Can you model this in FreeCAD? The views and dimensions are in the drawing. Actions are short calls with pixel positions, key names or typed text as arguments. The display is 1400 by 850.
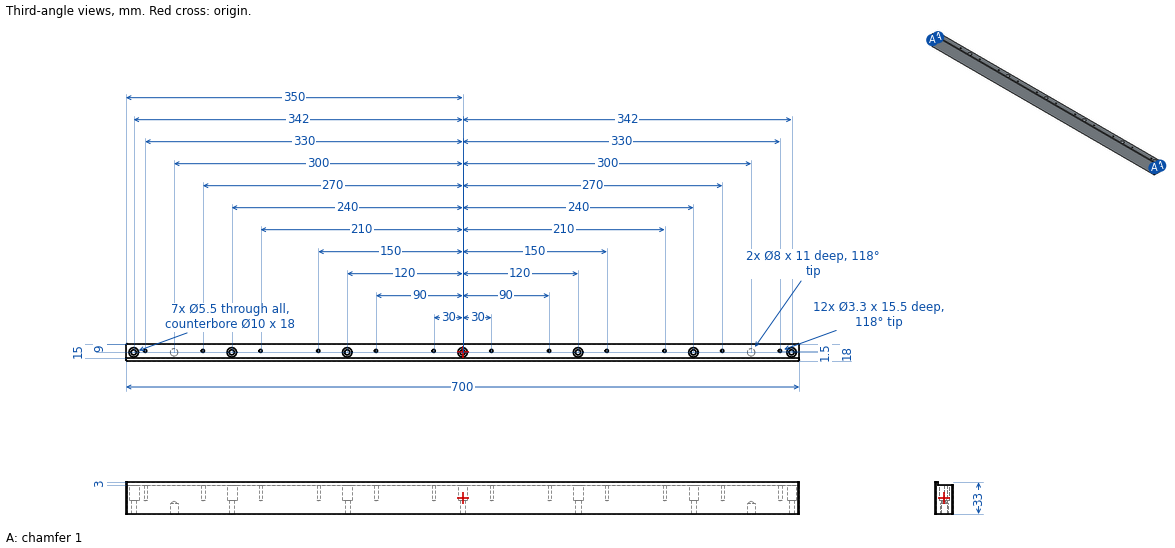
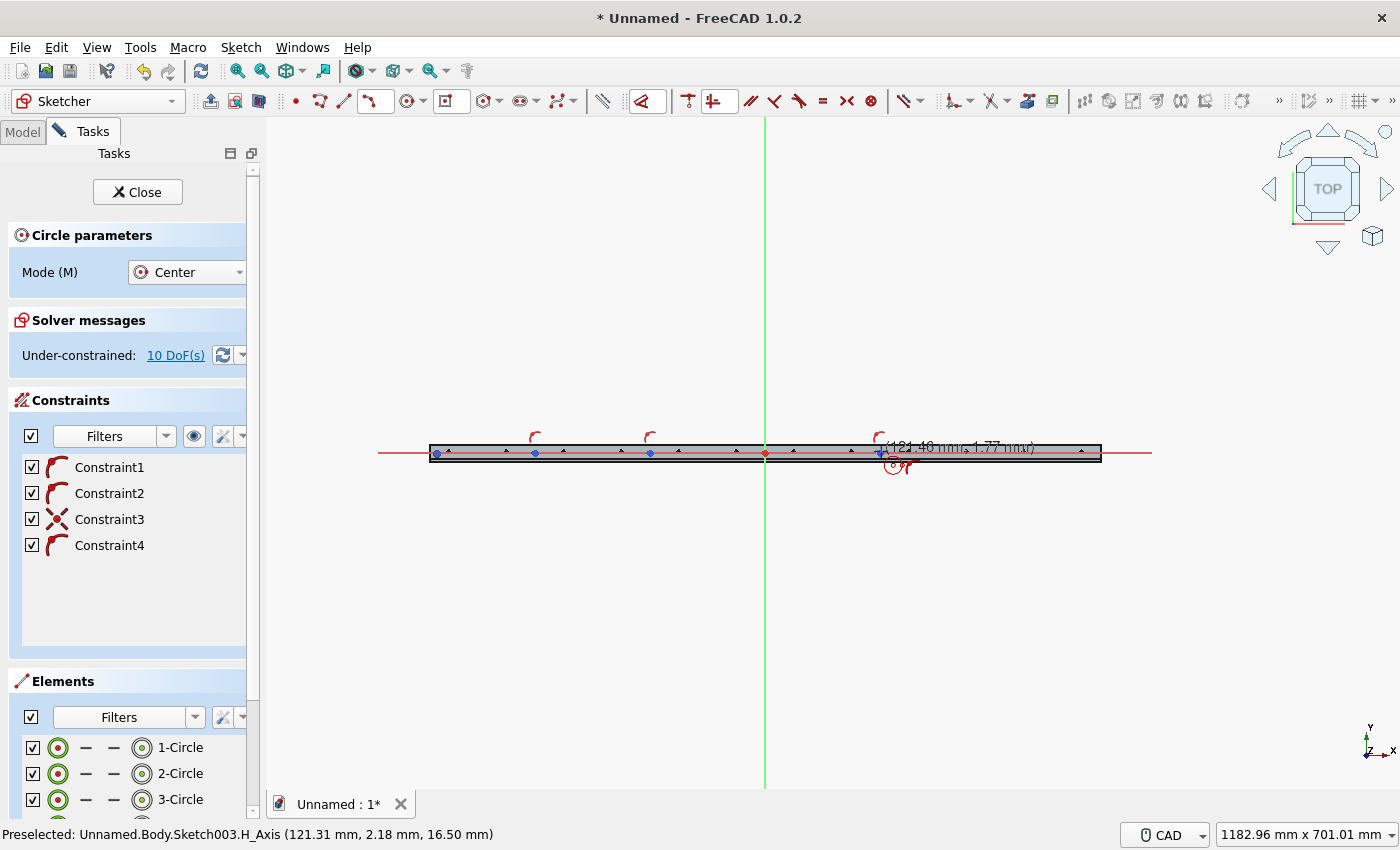
scroll(995, 453, up, 11)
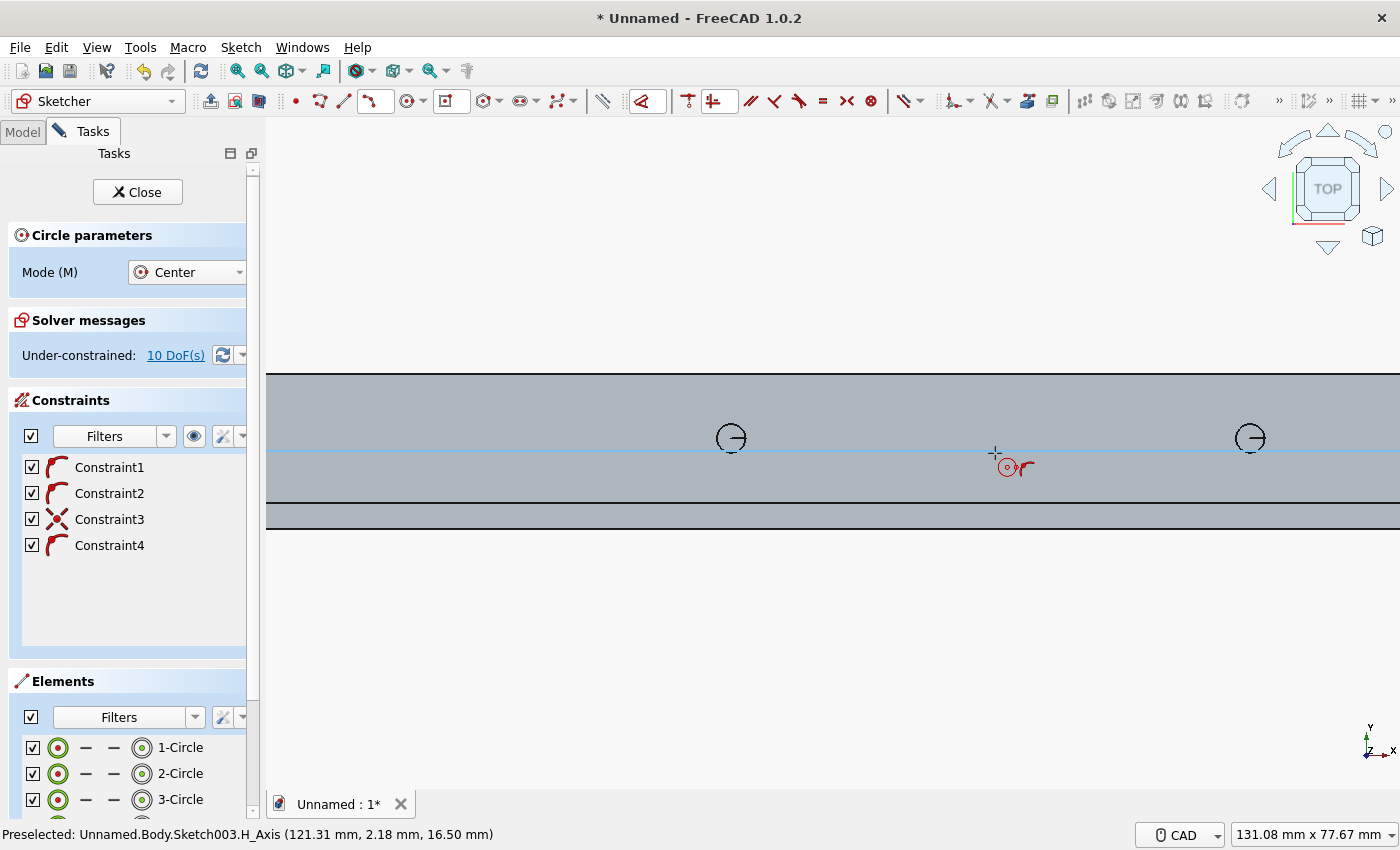
scroll(995, 453, down, 11)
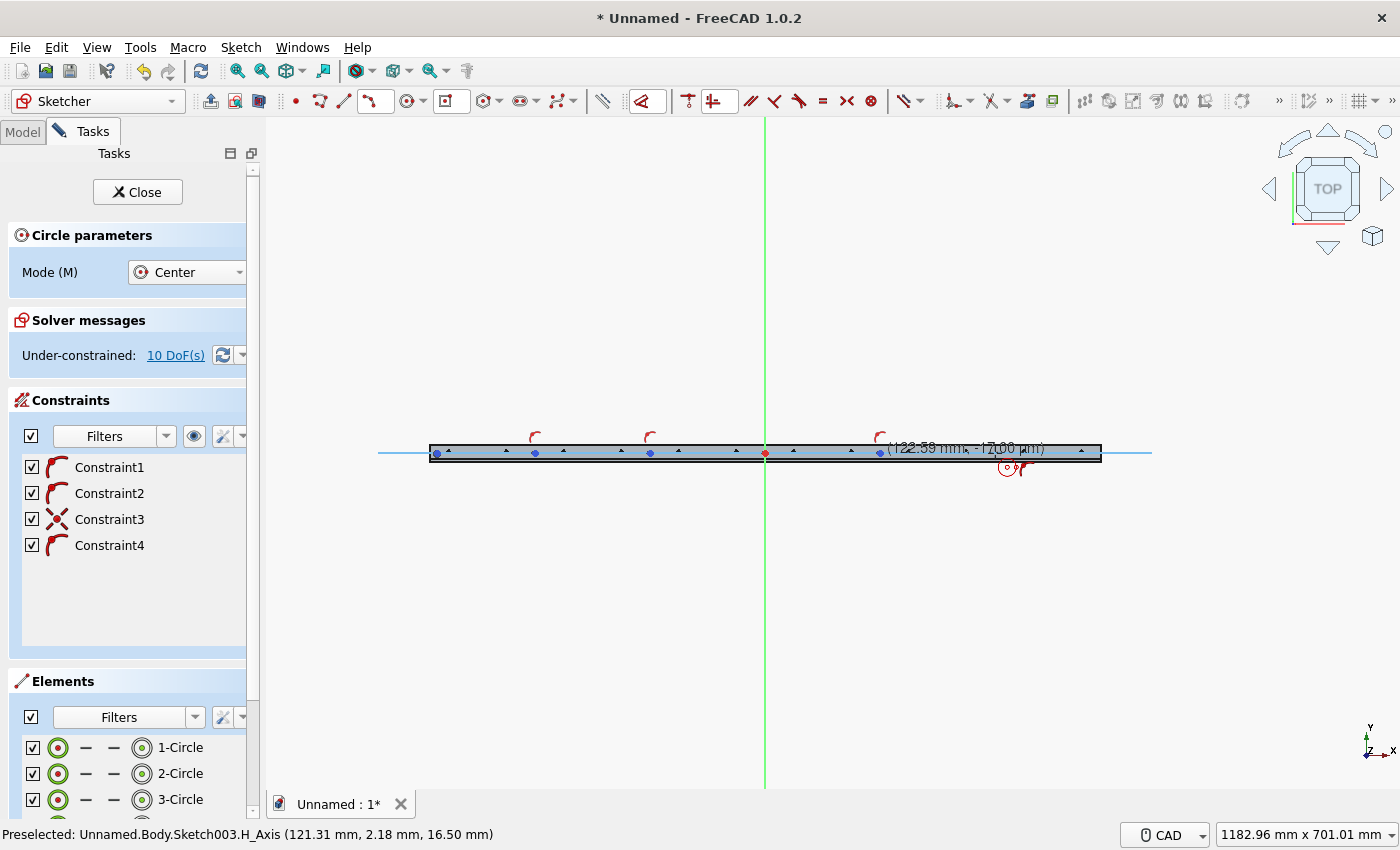
click(995, 453)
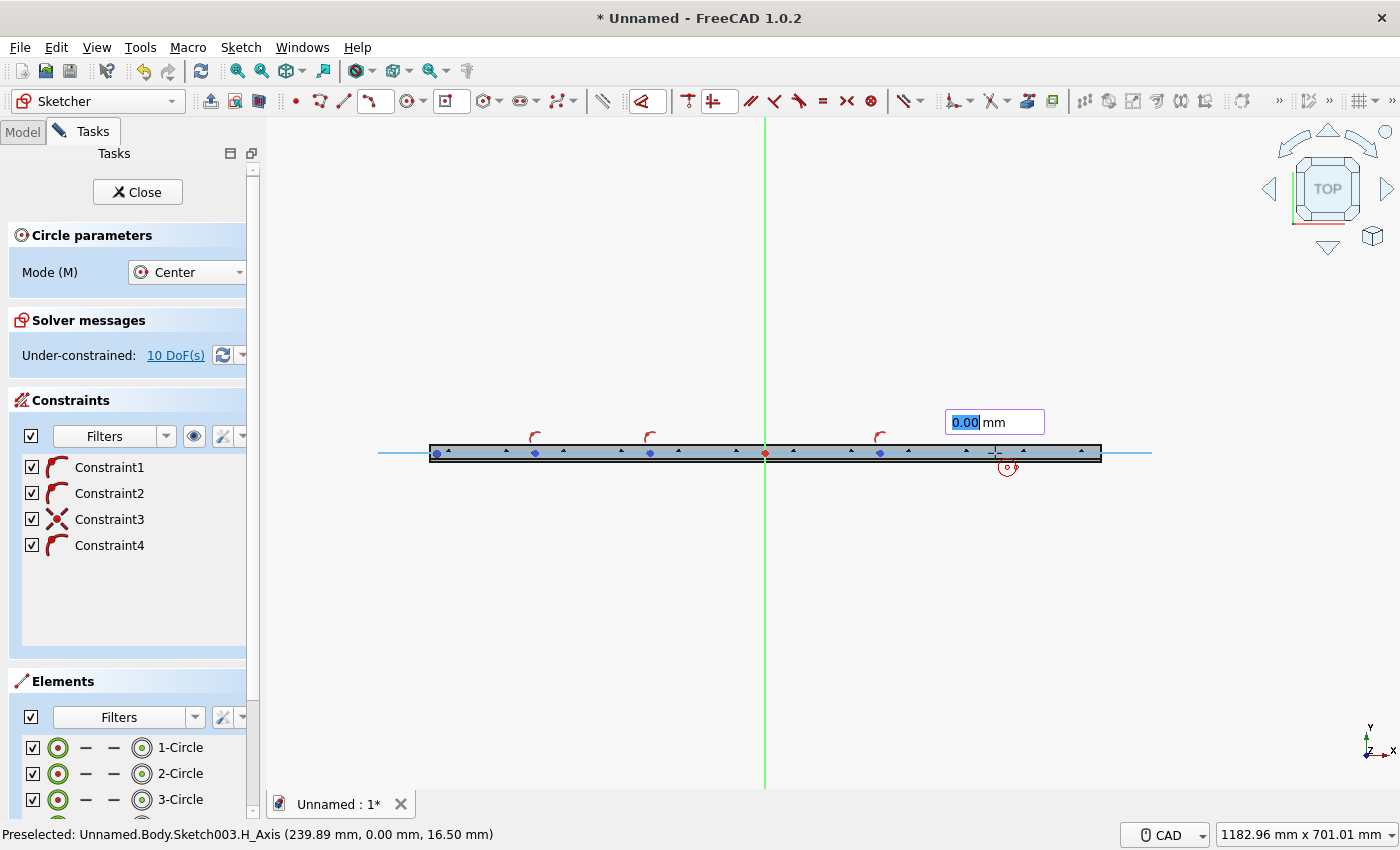
scroll(996, 451, up, 10)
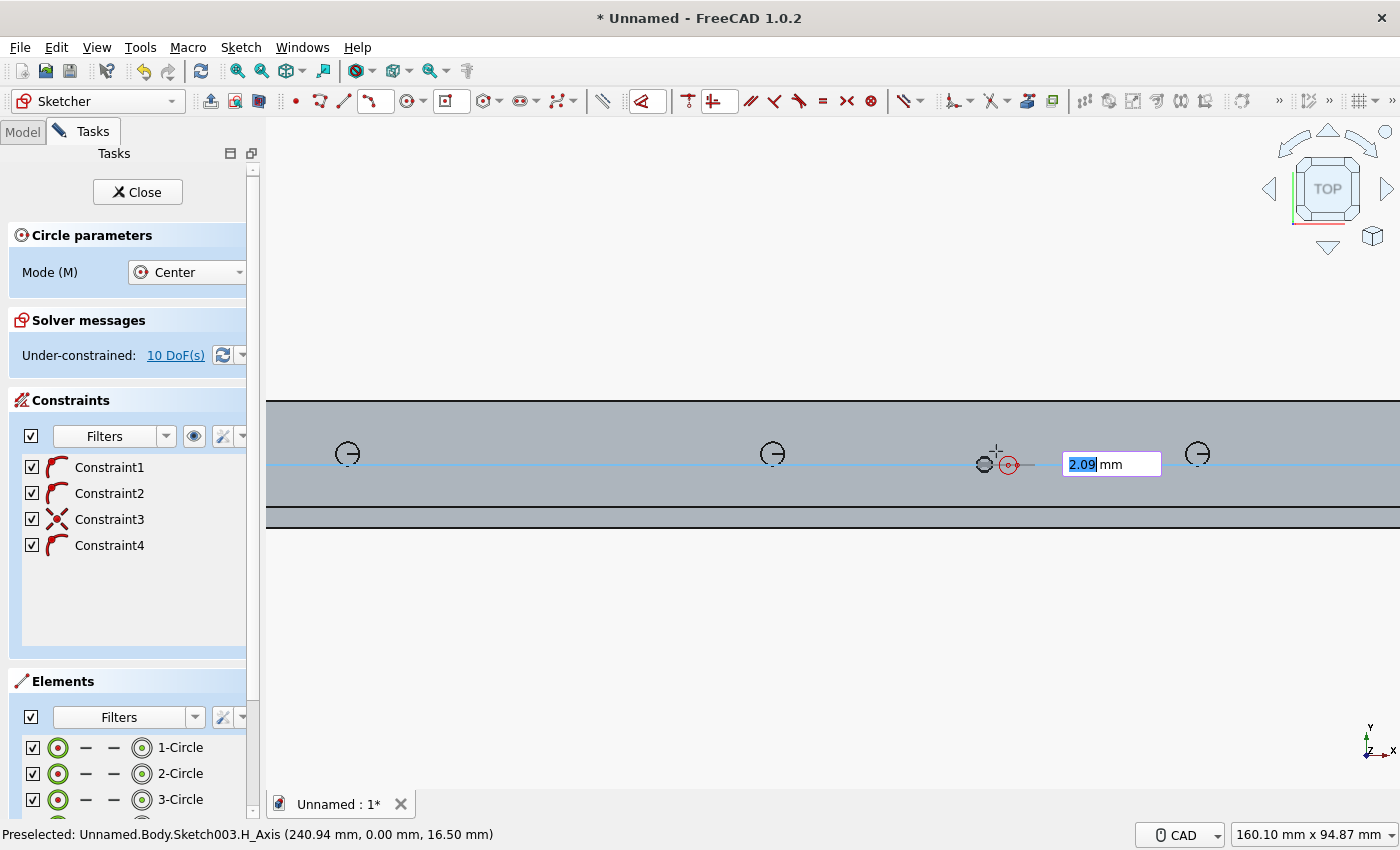
click(992, 446)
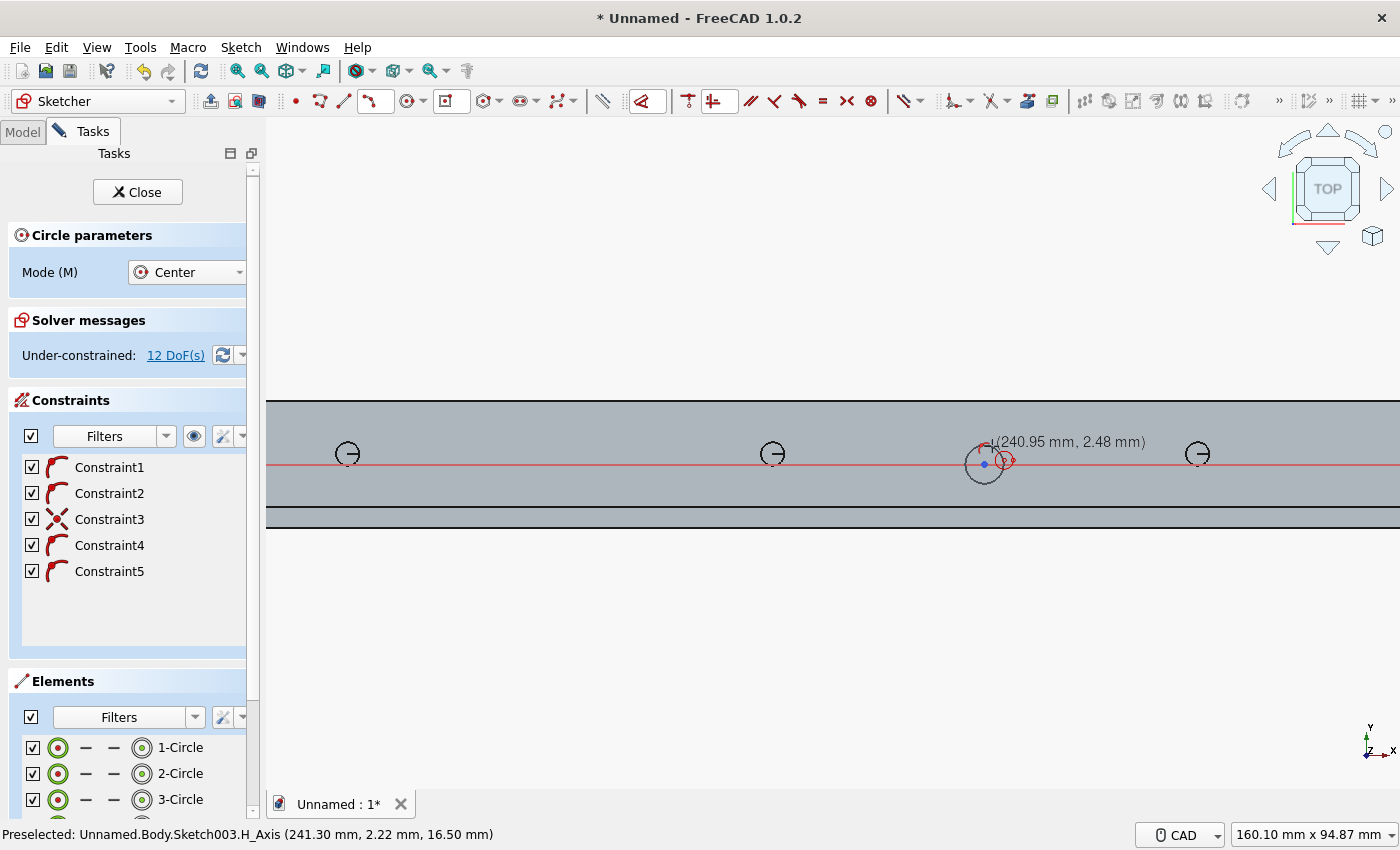
scroll(996, 451, down, 10)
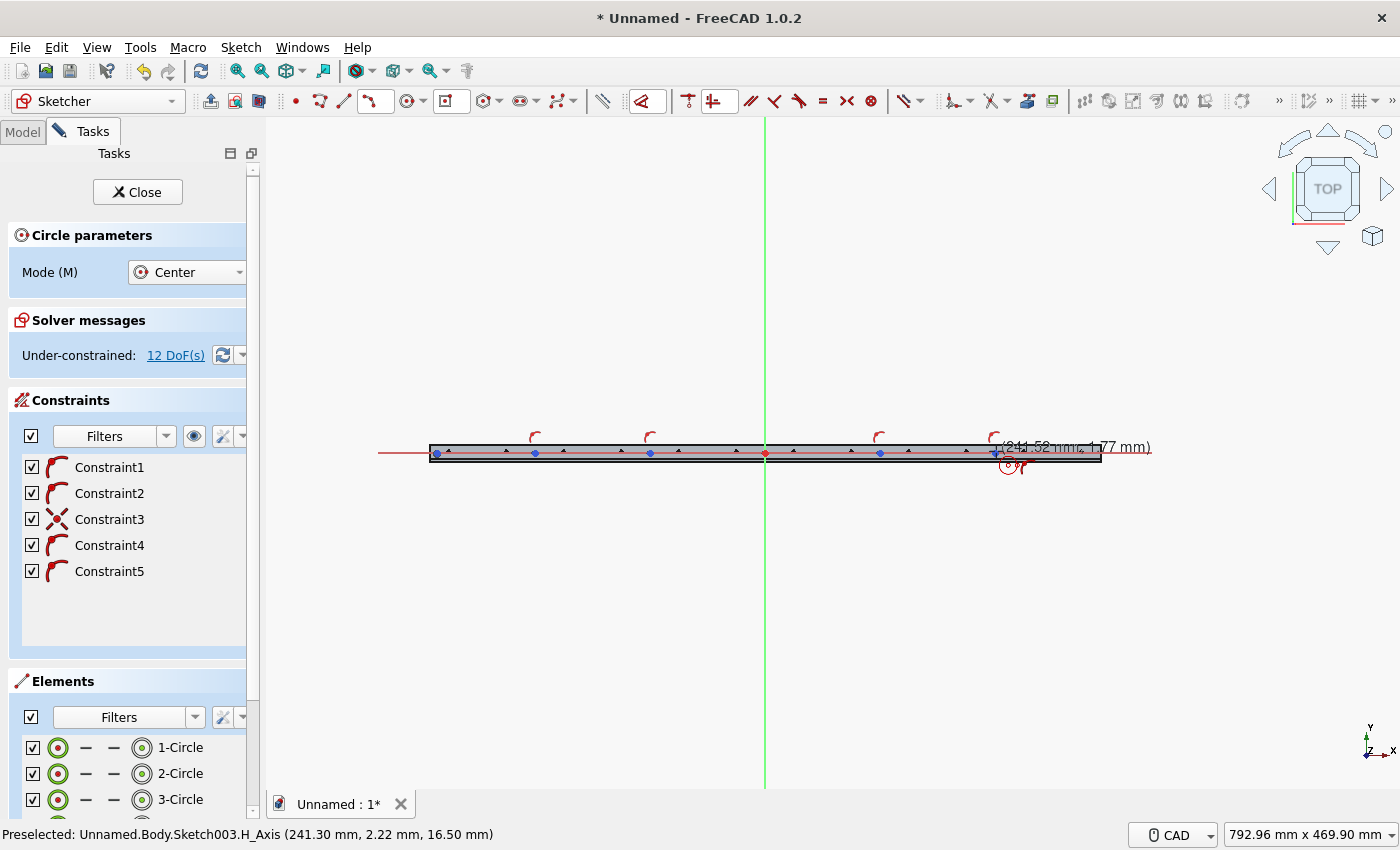
scroll(1093, 453, up, 11)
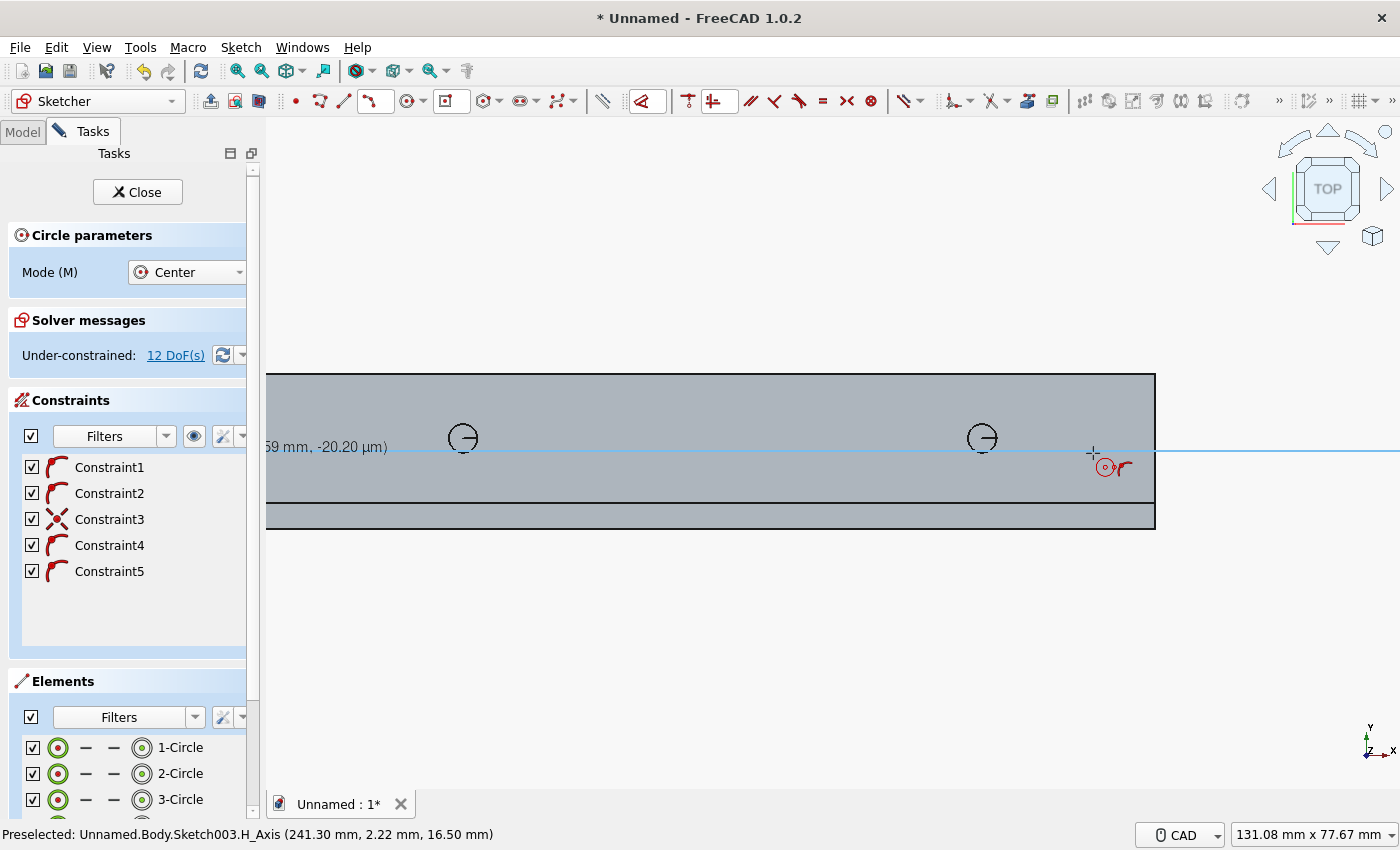
scroll(1093, 453, down, 11)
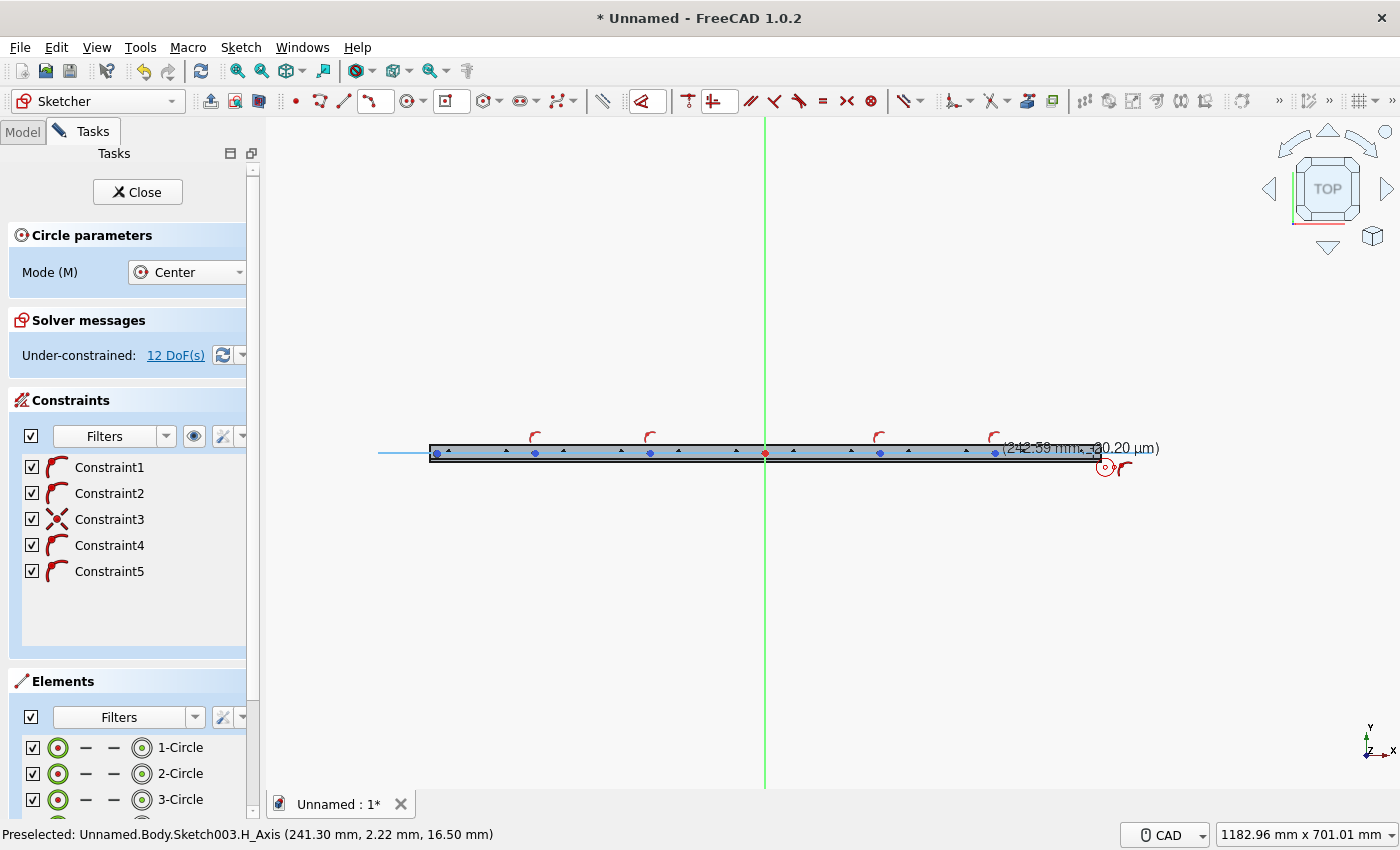
click(1093, 453)